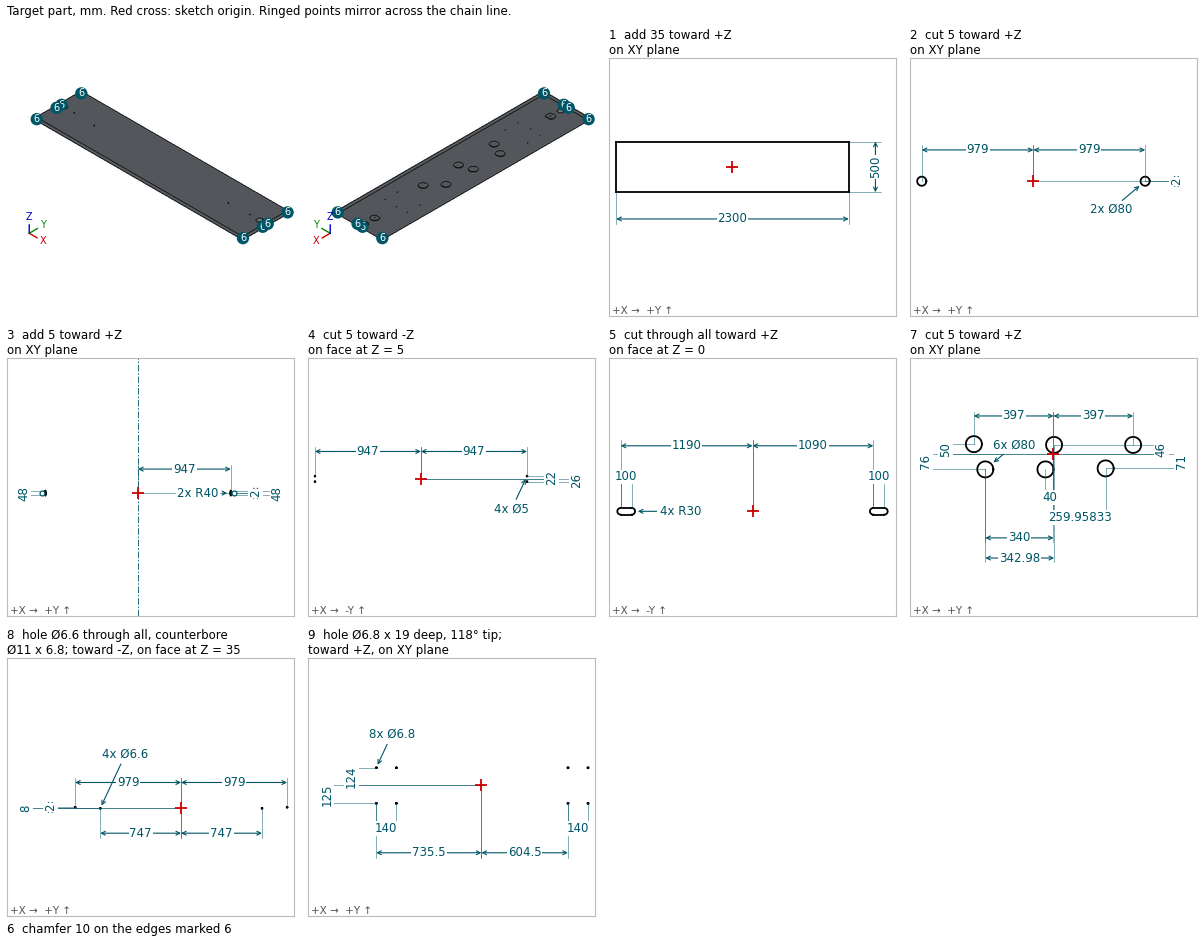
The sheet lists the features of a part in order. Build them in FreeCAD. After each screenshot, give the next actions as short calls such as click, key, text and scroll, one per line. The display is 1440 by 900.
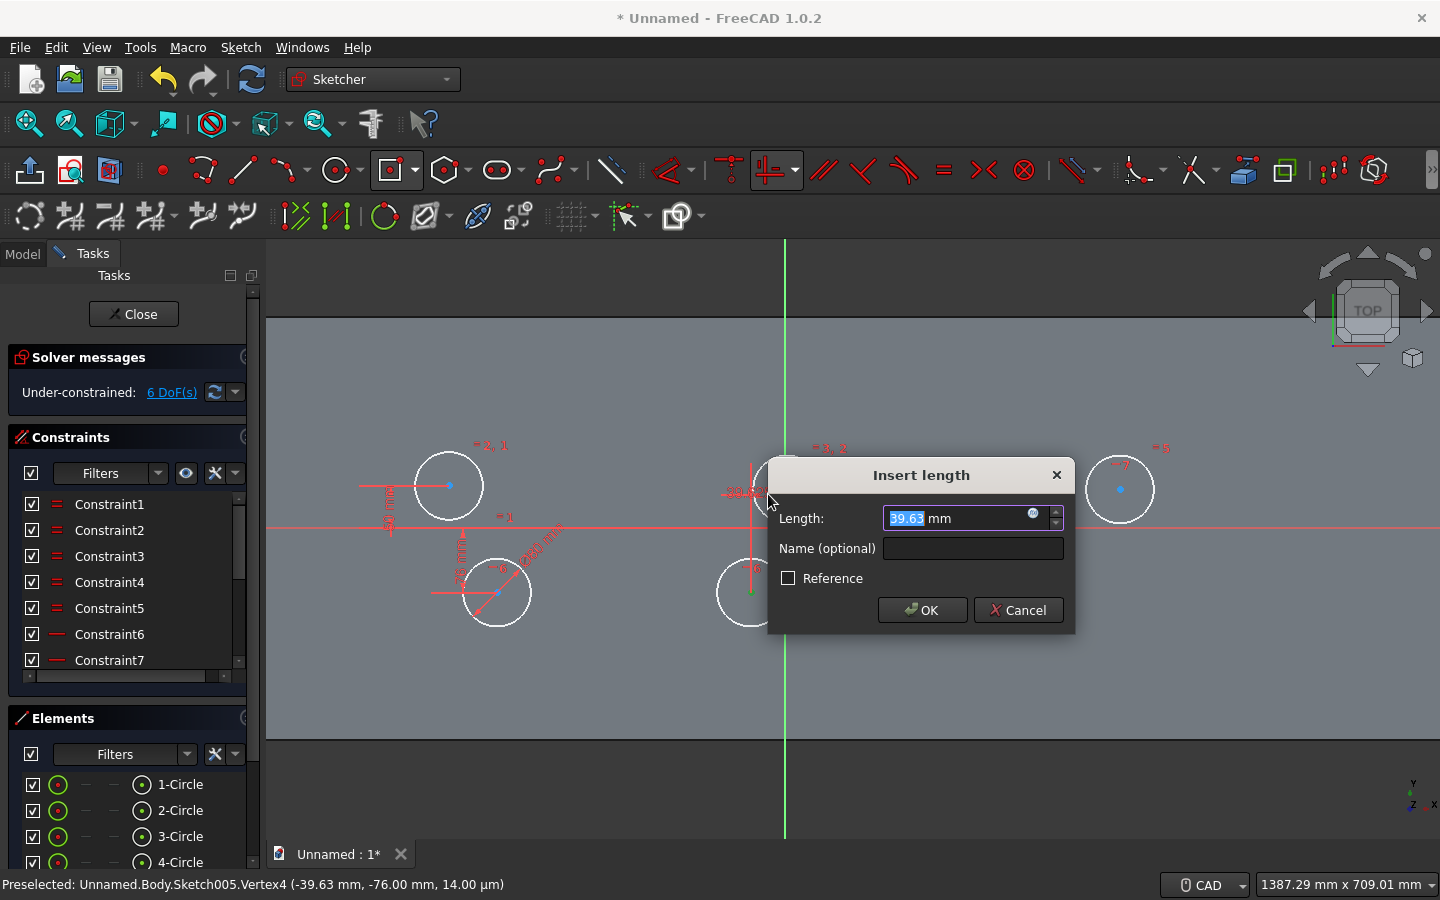
text(40)
key(Return)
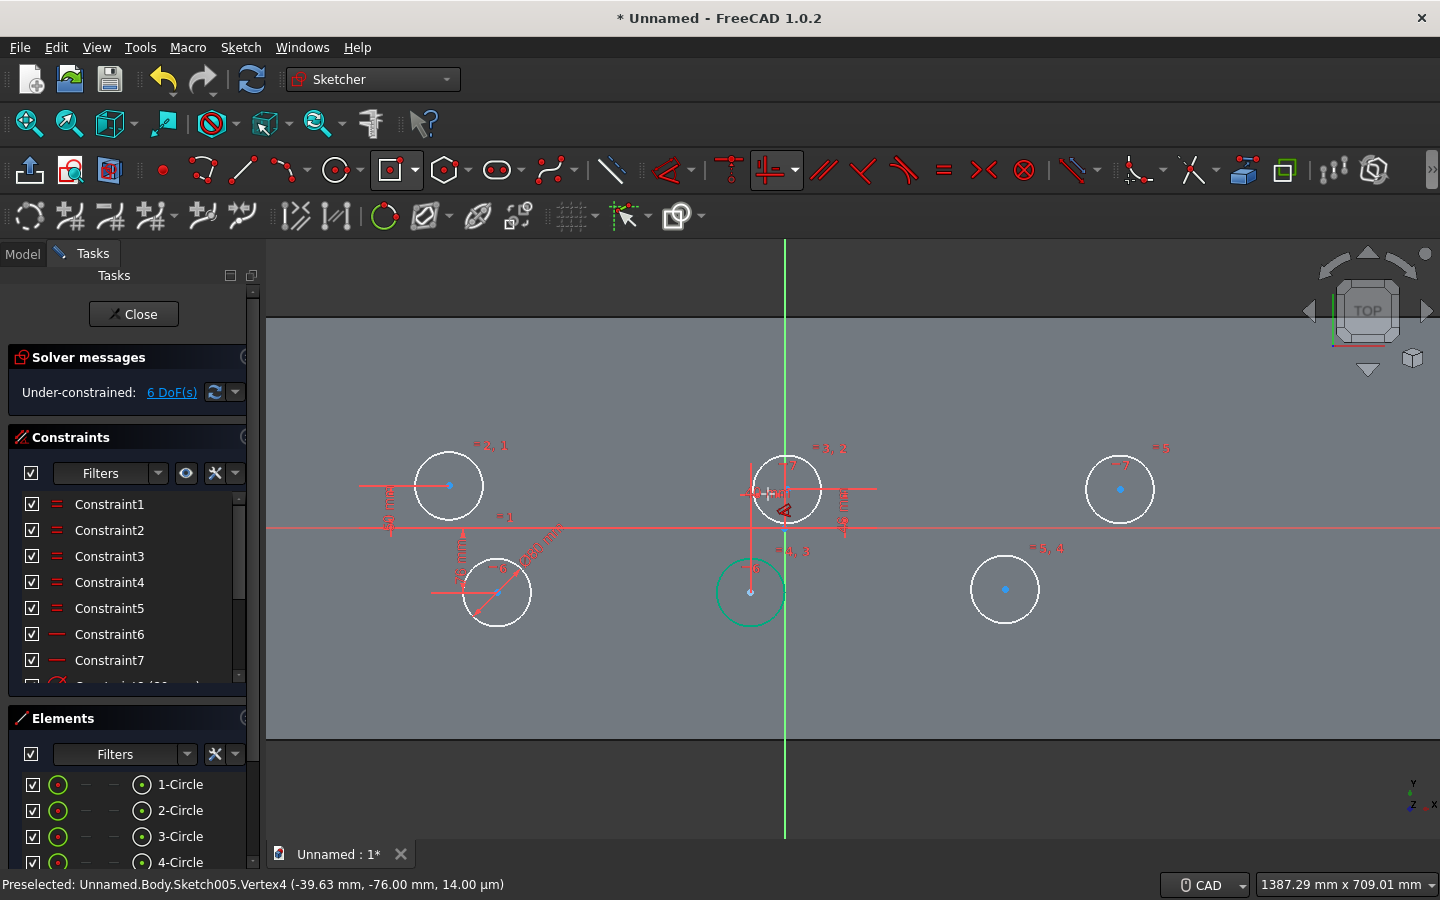
click(1005, 589)
click(1039, 545)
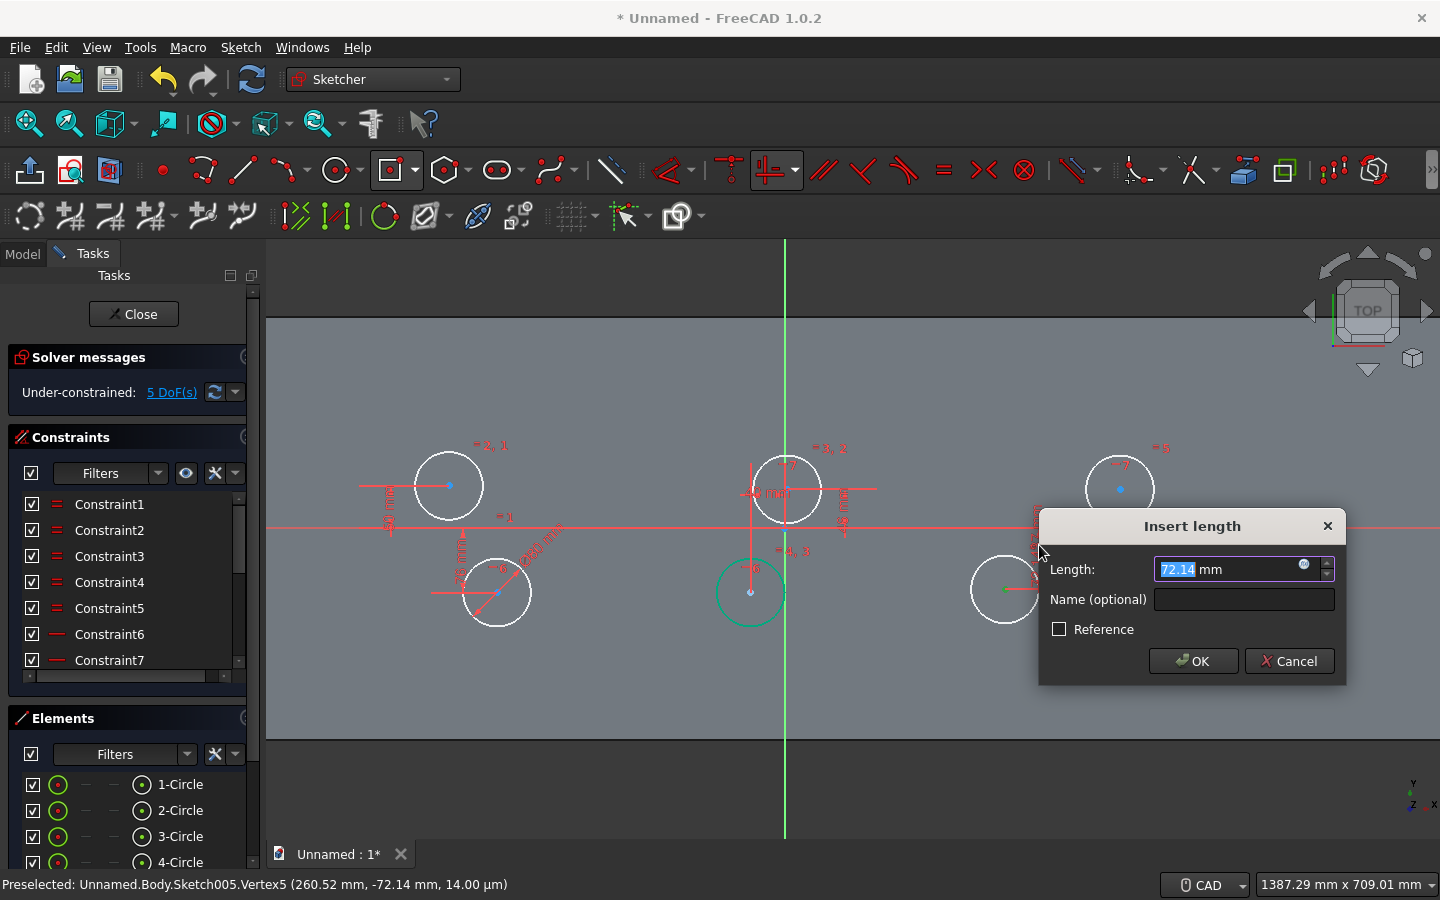
text(71)
key(Return)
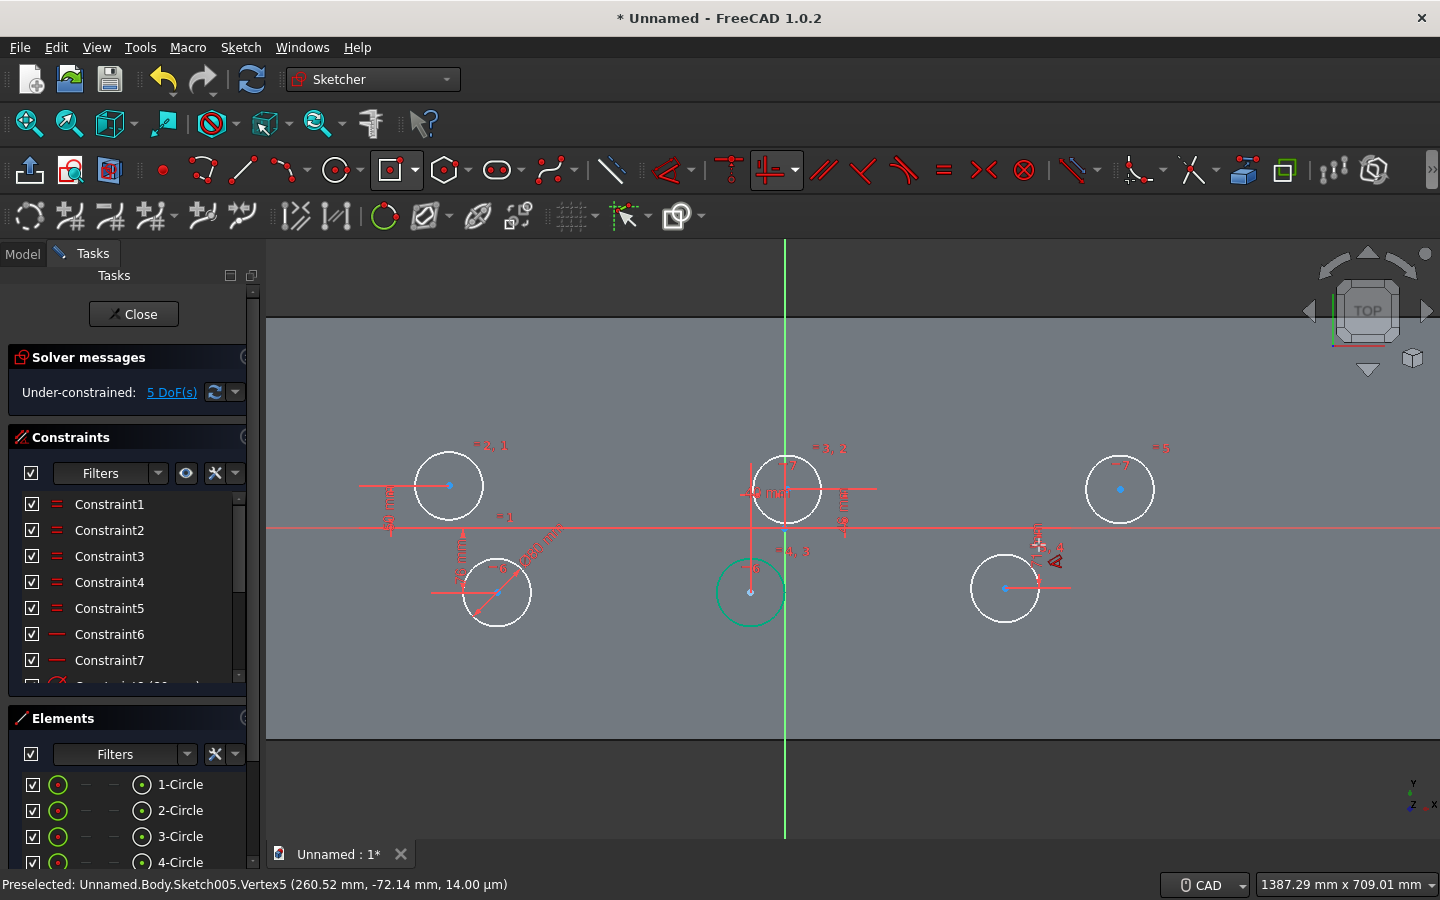
click(497, 593)
click(641, 627)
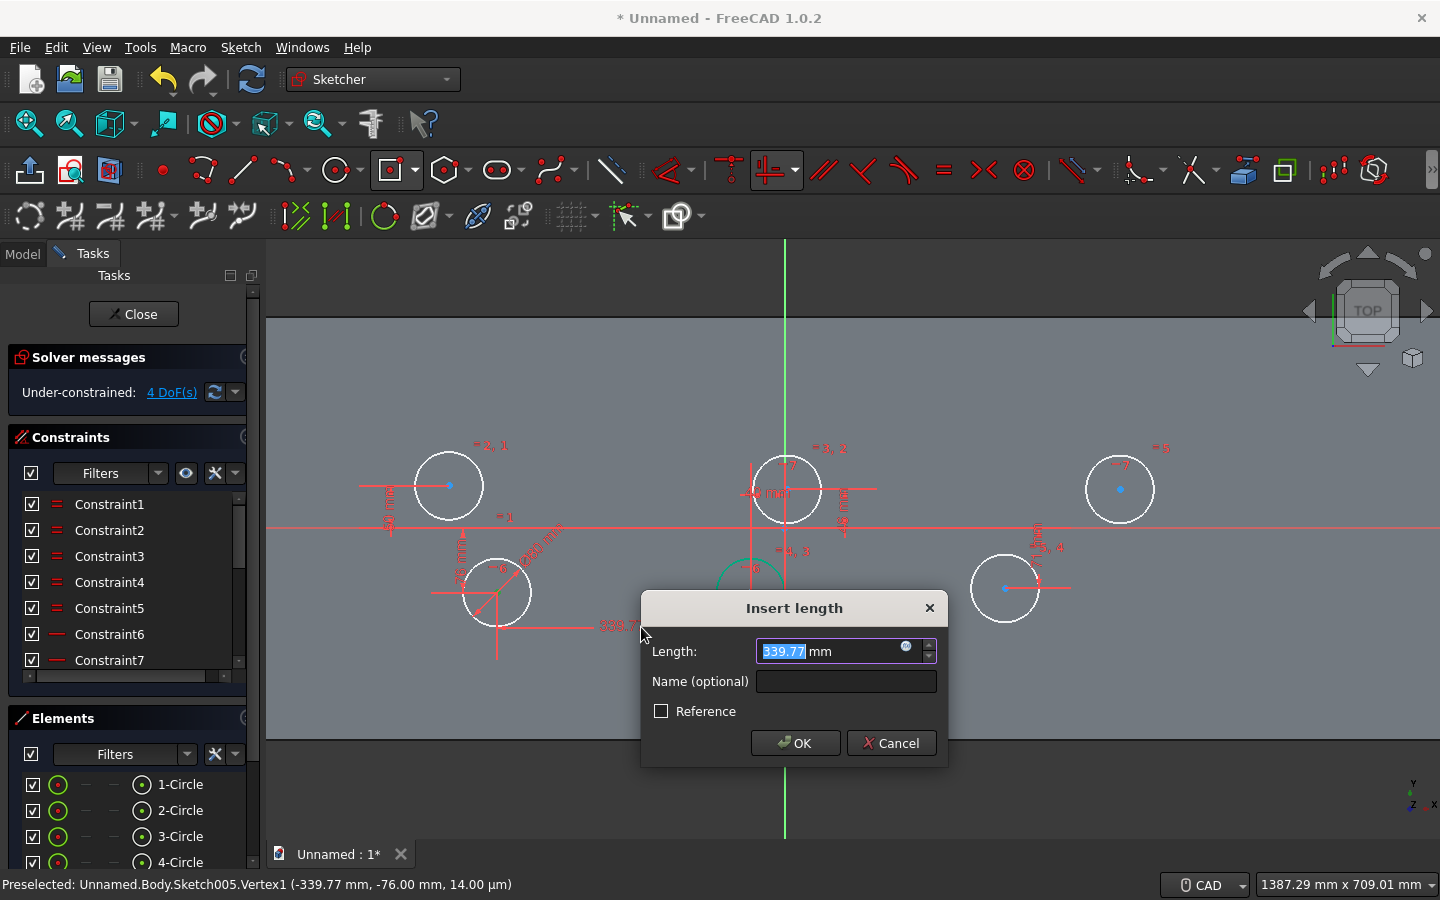
text(340)
key(Return)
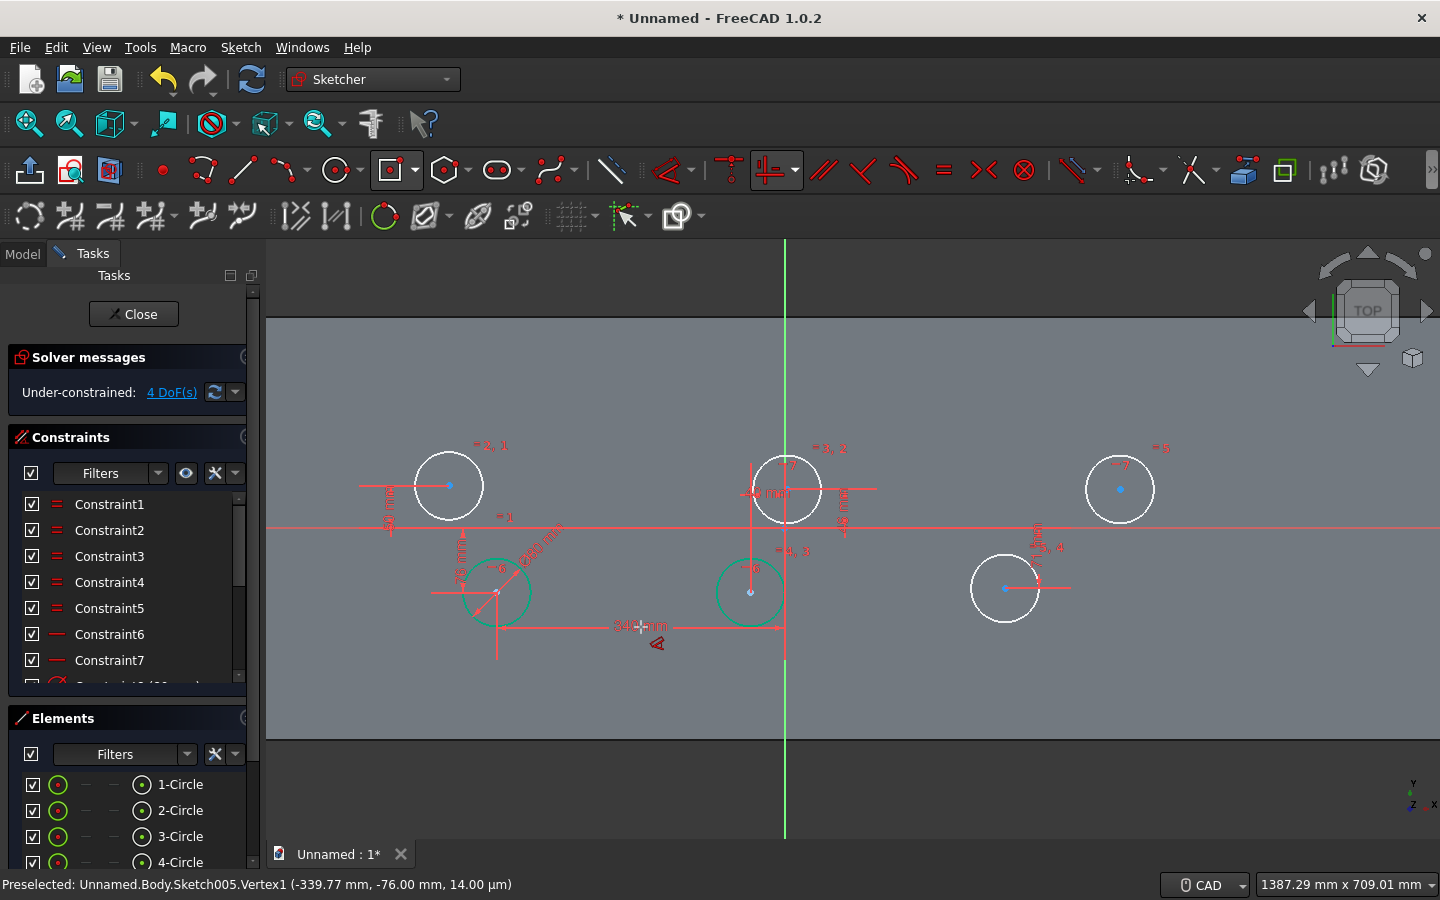
click(449, 486)
click(617, 452)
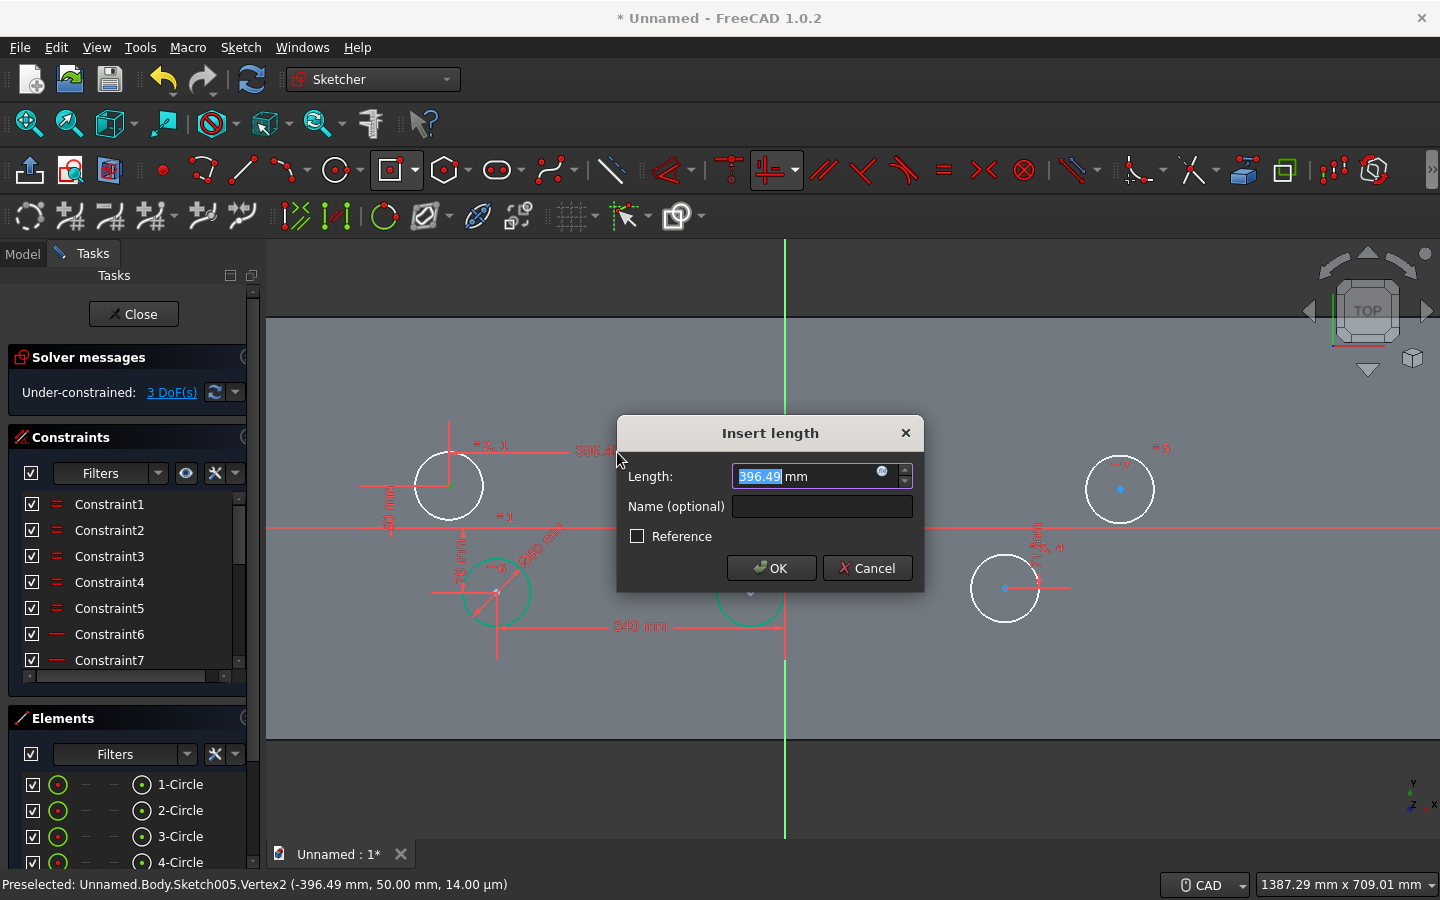
text(397)
key(Return)